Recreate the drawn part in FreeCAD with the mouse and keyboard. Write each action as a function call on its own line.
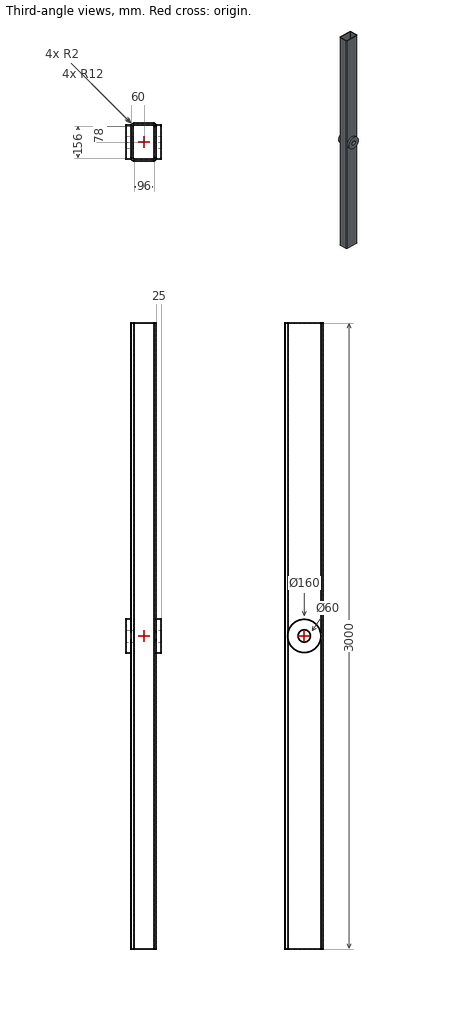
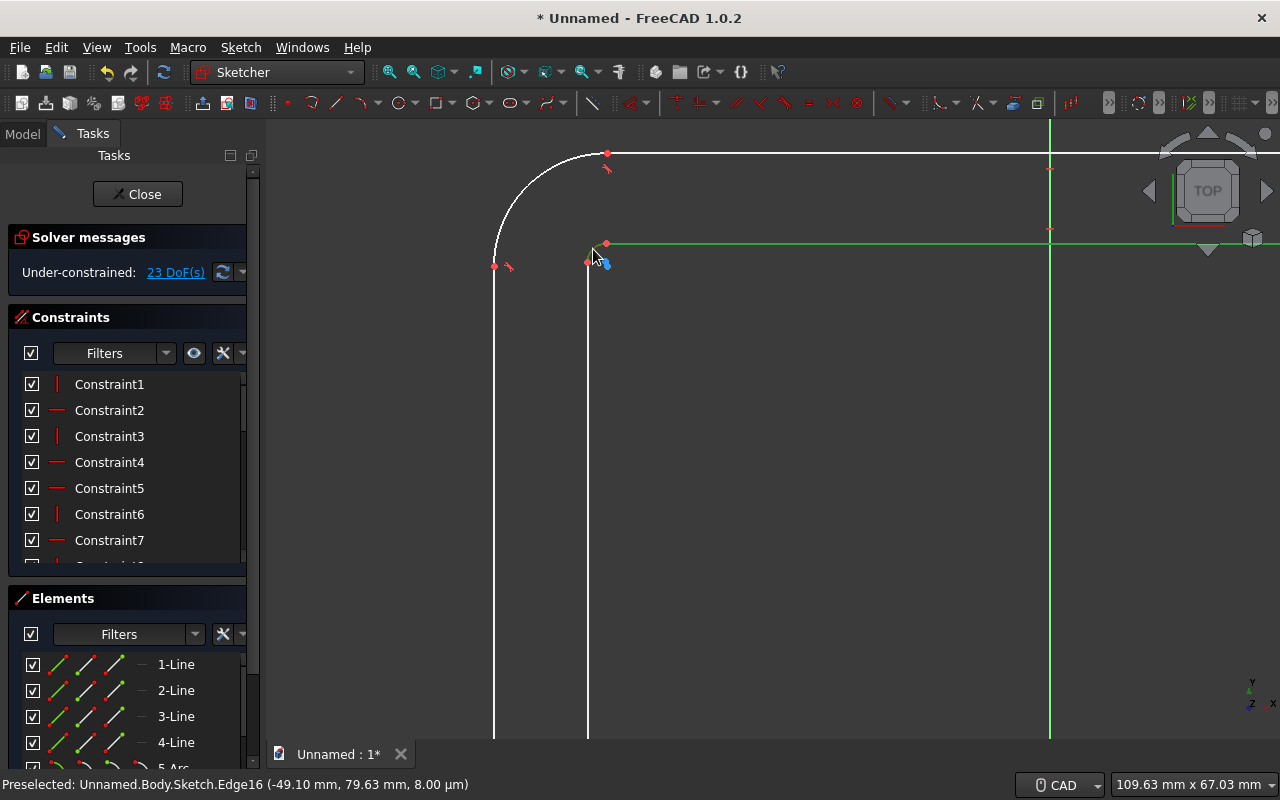
click(786, 104)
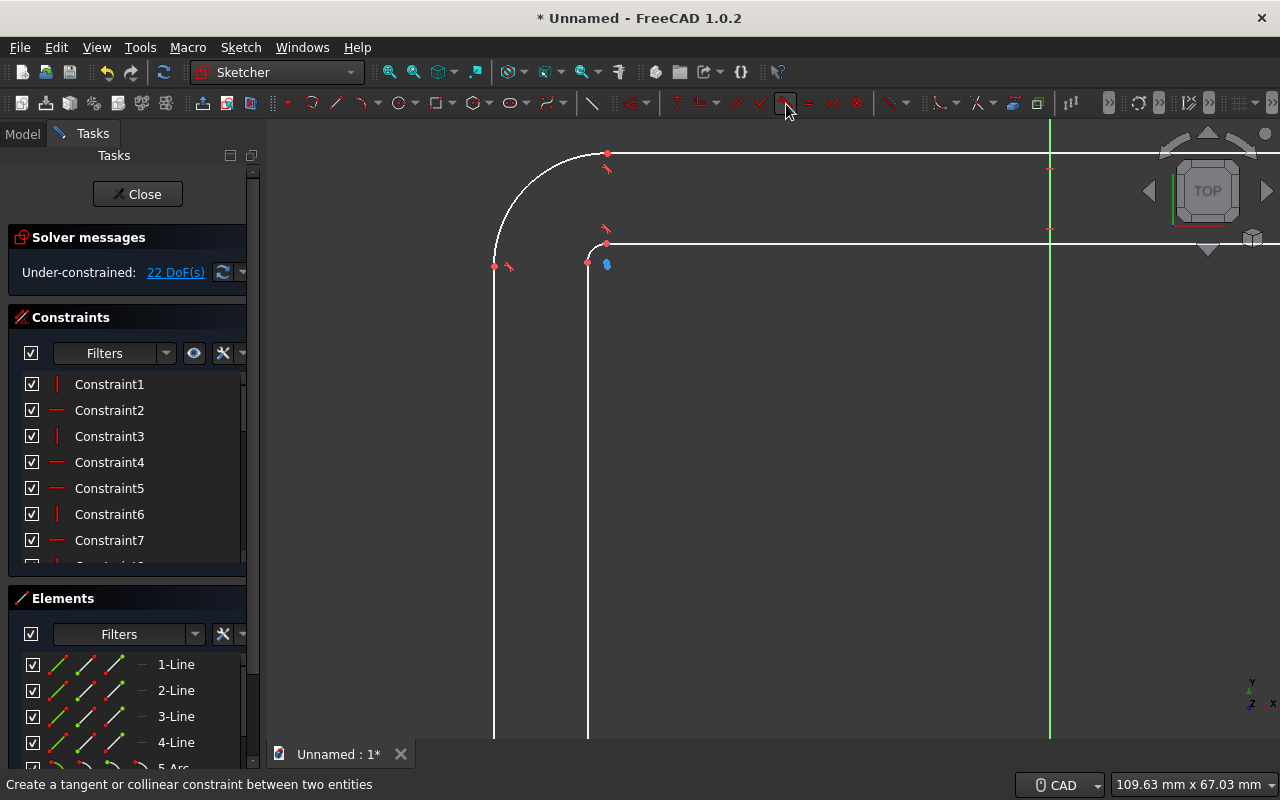
scroll(591, 248, down, 7)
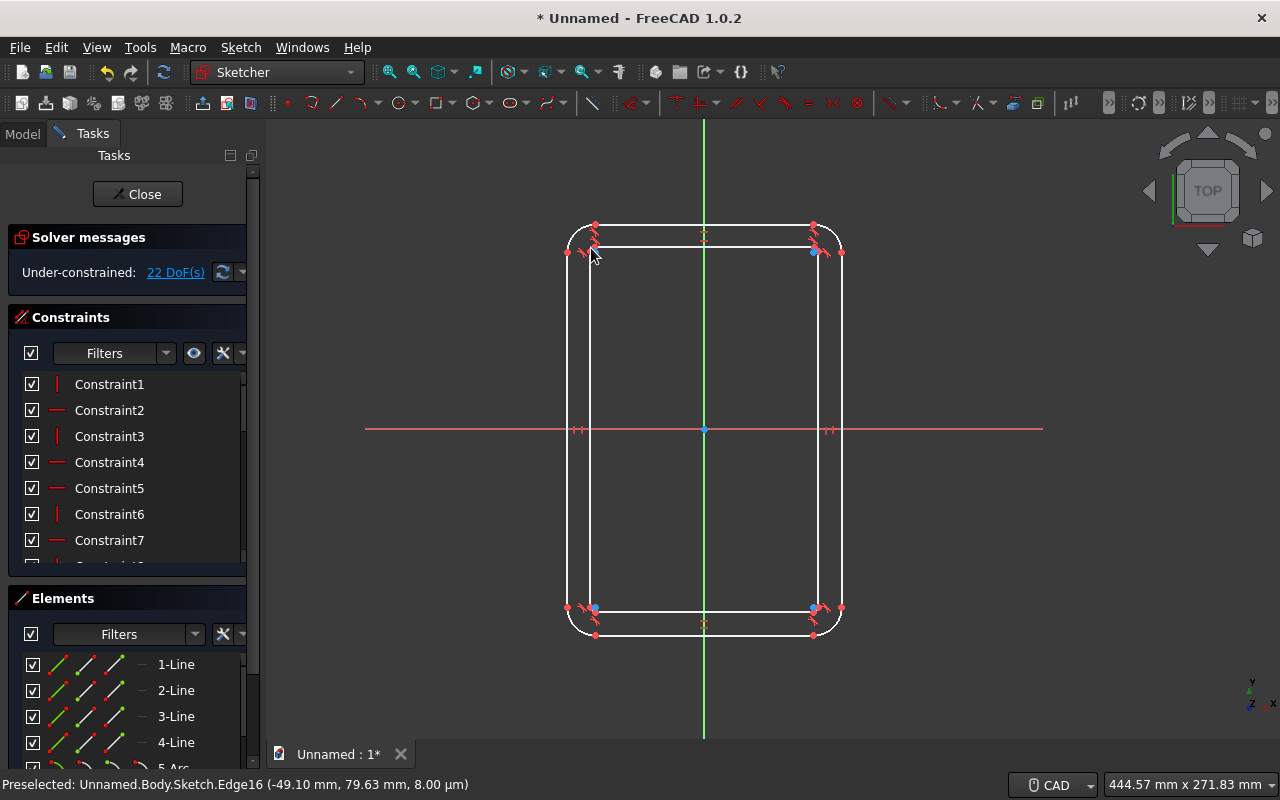
click(818, 359)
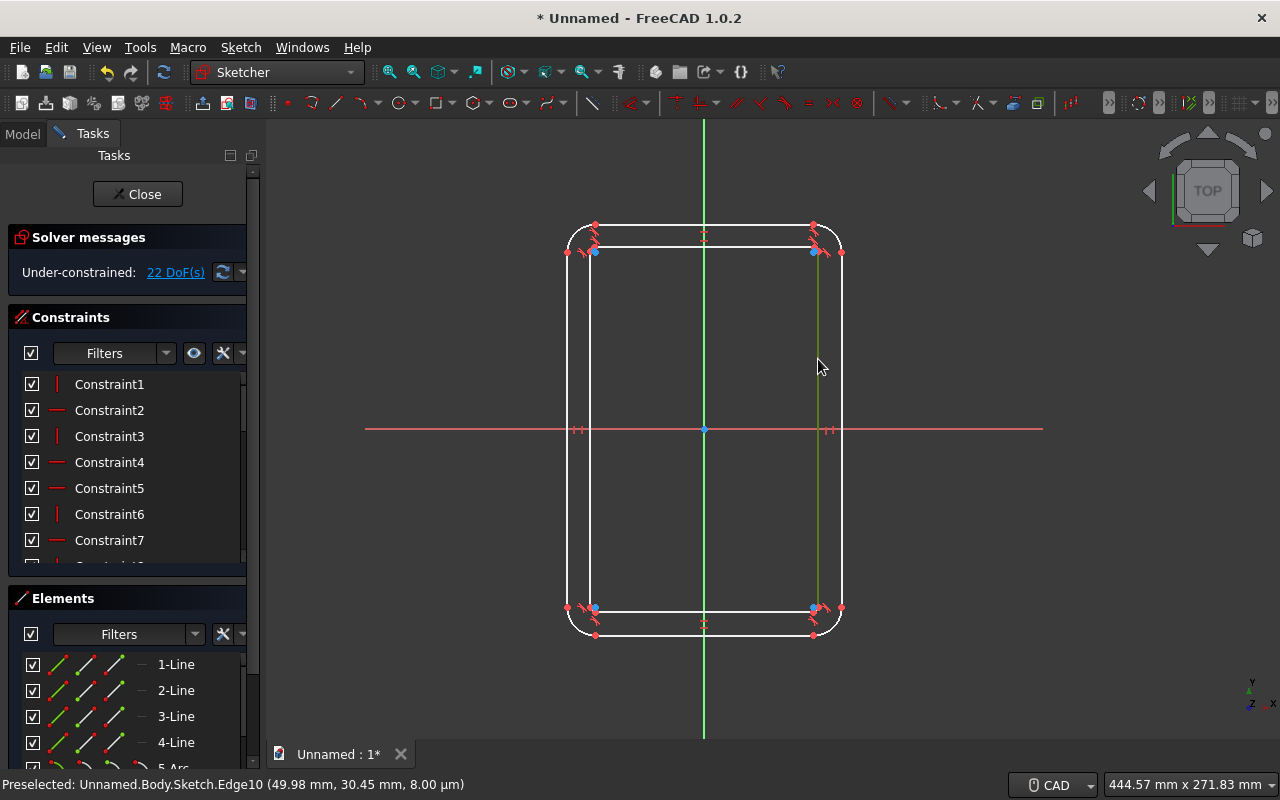
scroll(817, 249, up, 7)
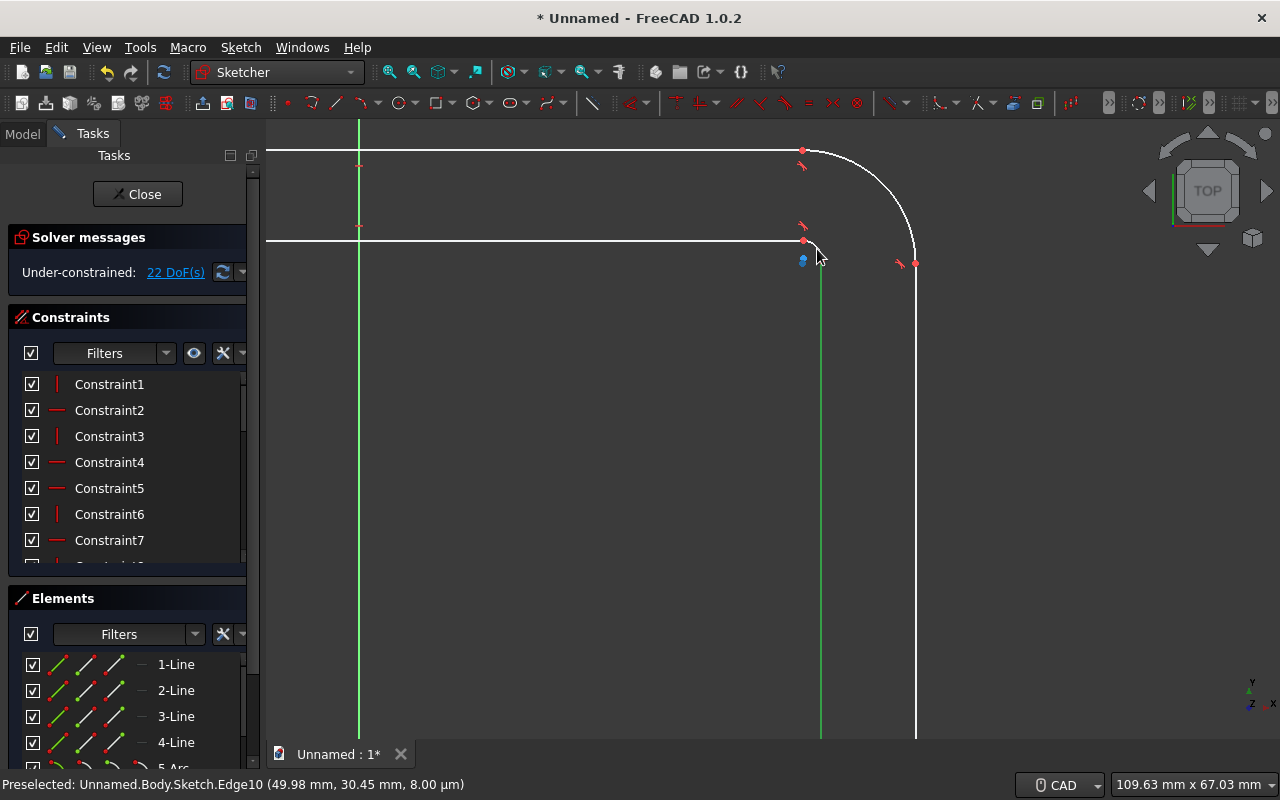
click(816, 247)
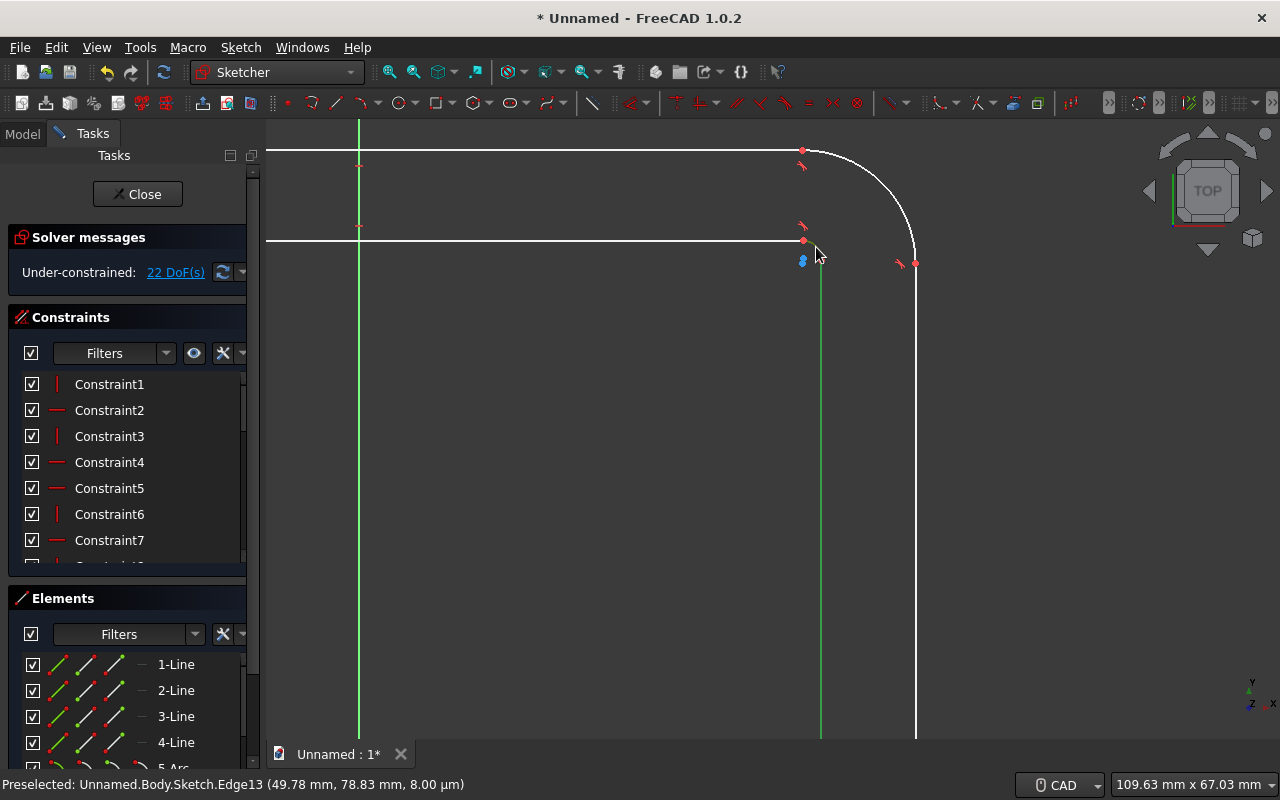
click(786, 104)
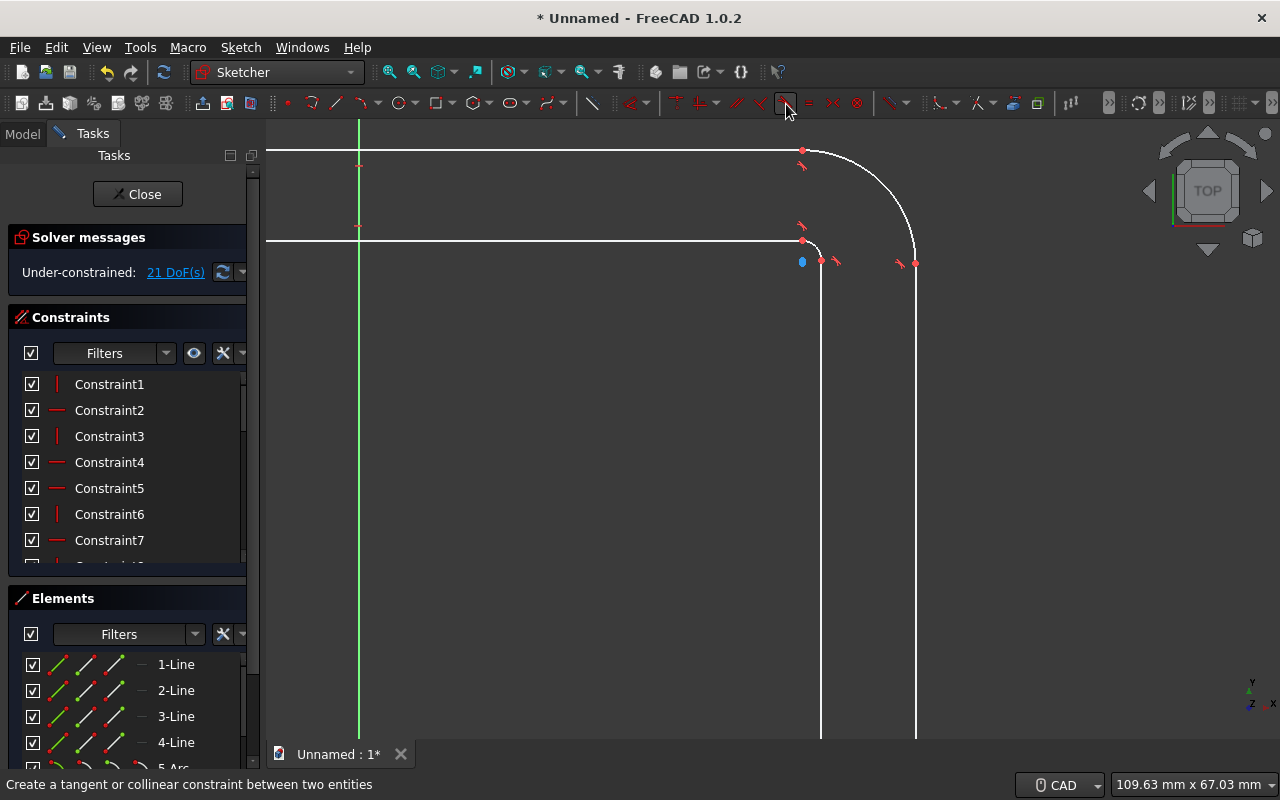
scroll(818, 249, down, 7)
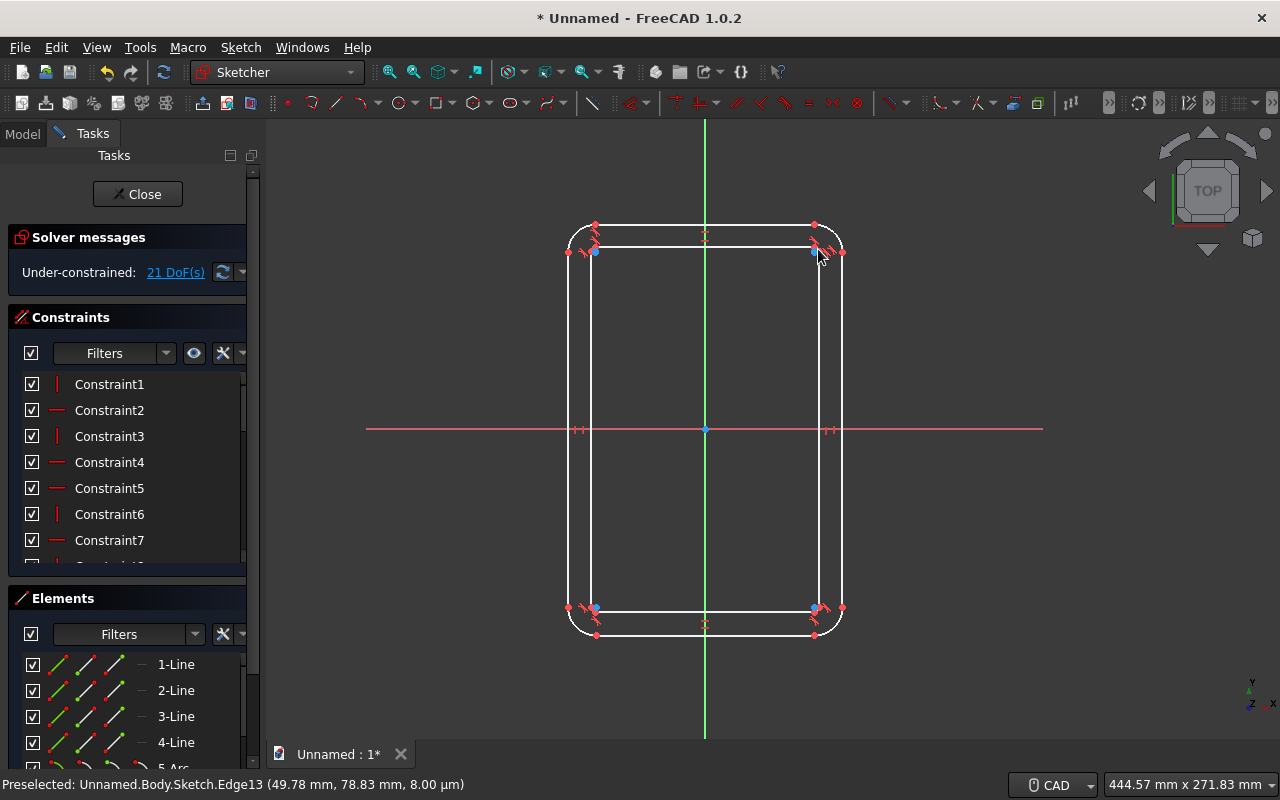
click(819, 359)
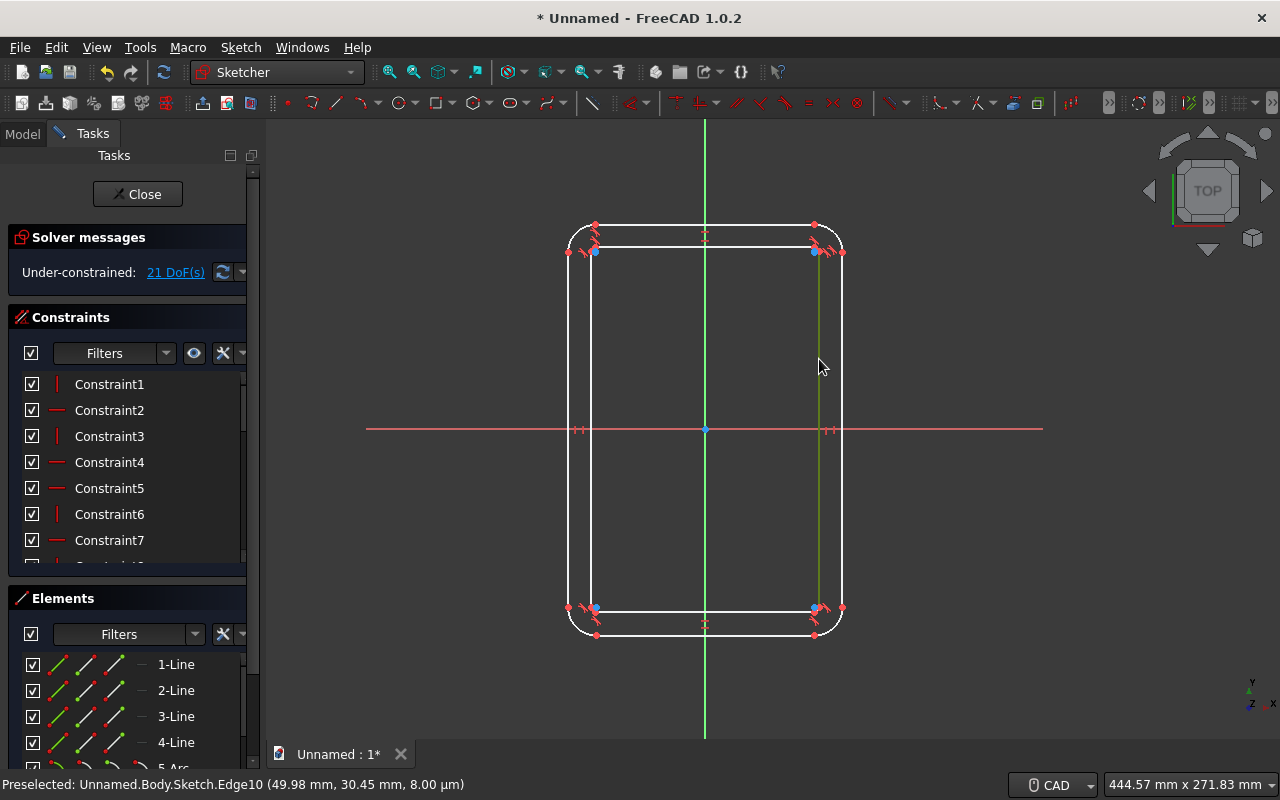
scroll(818, 611, up, 7)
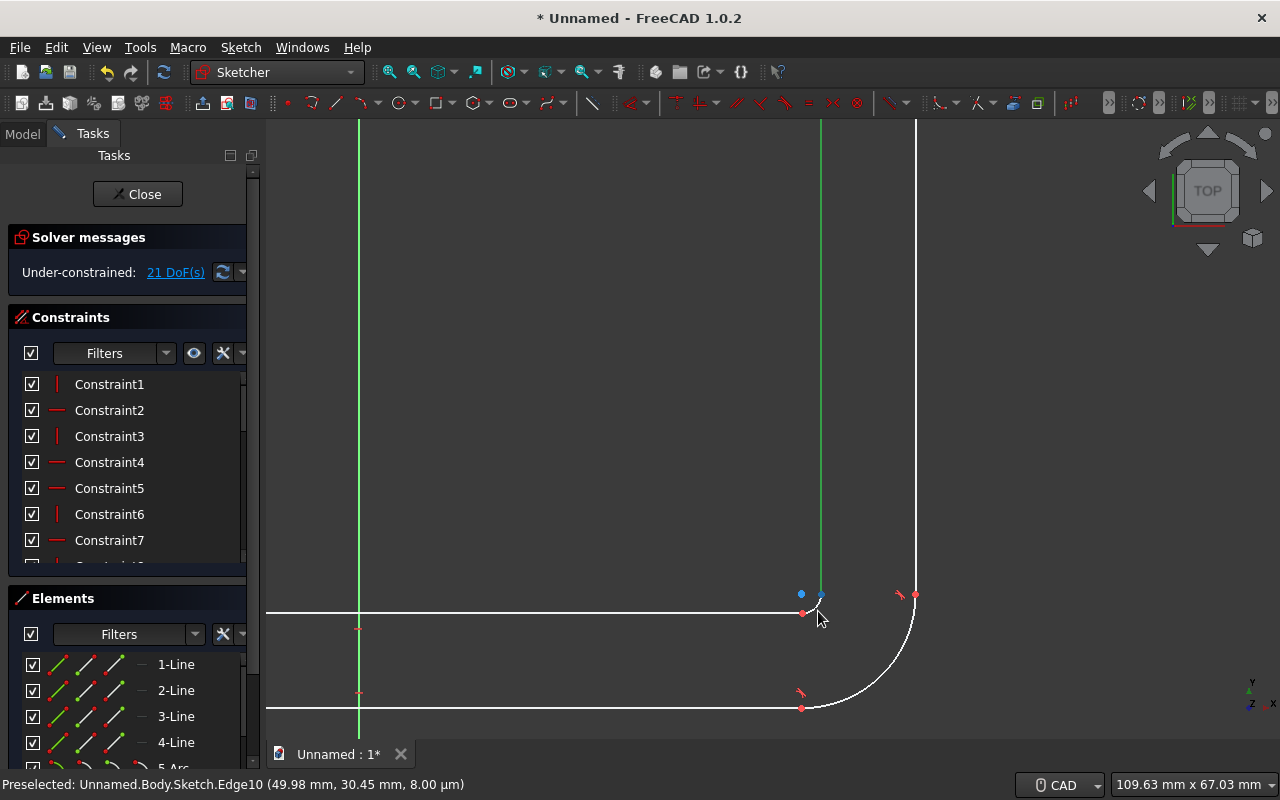
click(816, 608)